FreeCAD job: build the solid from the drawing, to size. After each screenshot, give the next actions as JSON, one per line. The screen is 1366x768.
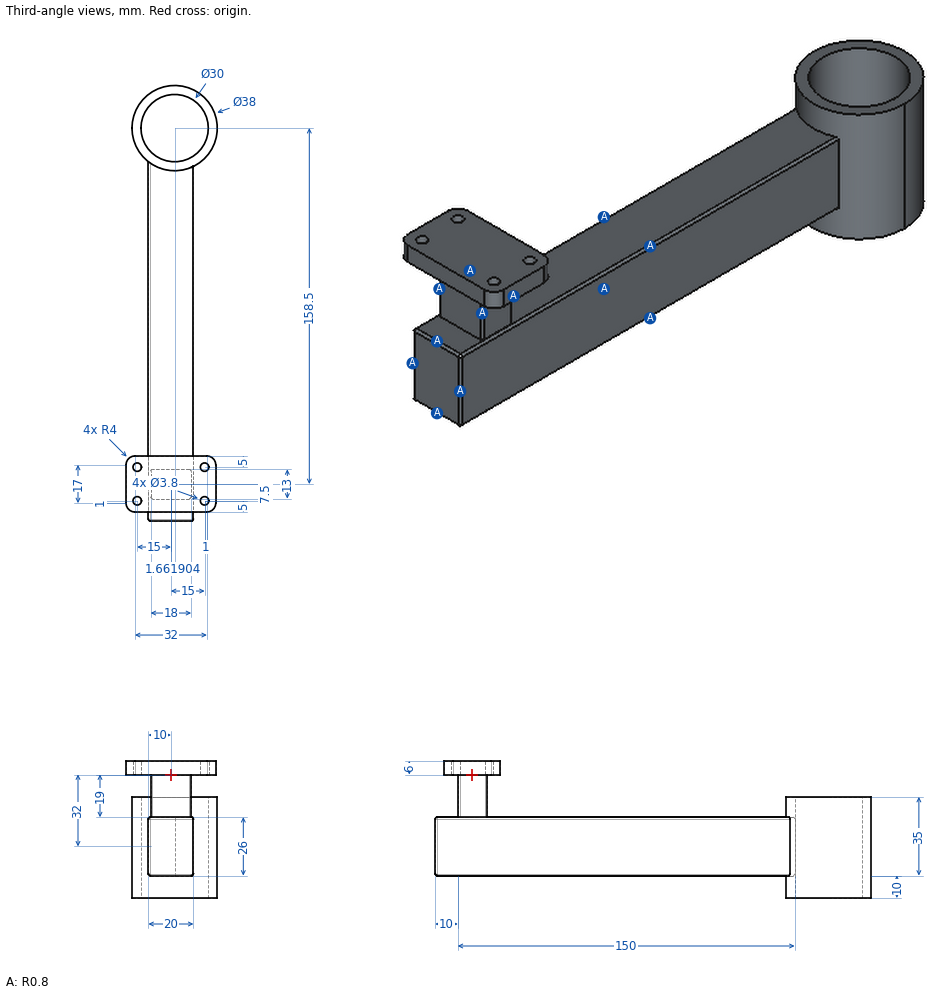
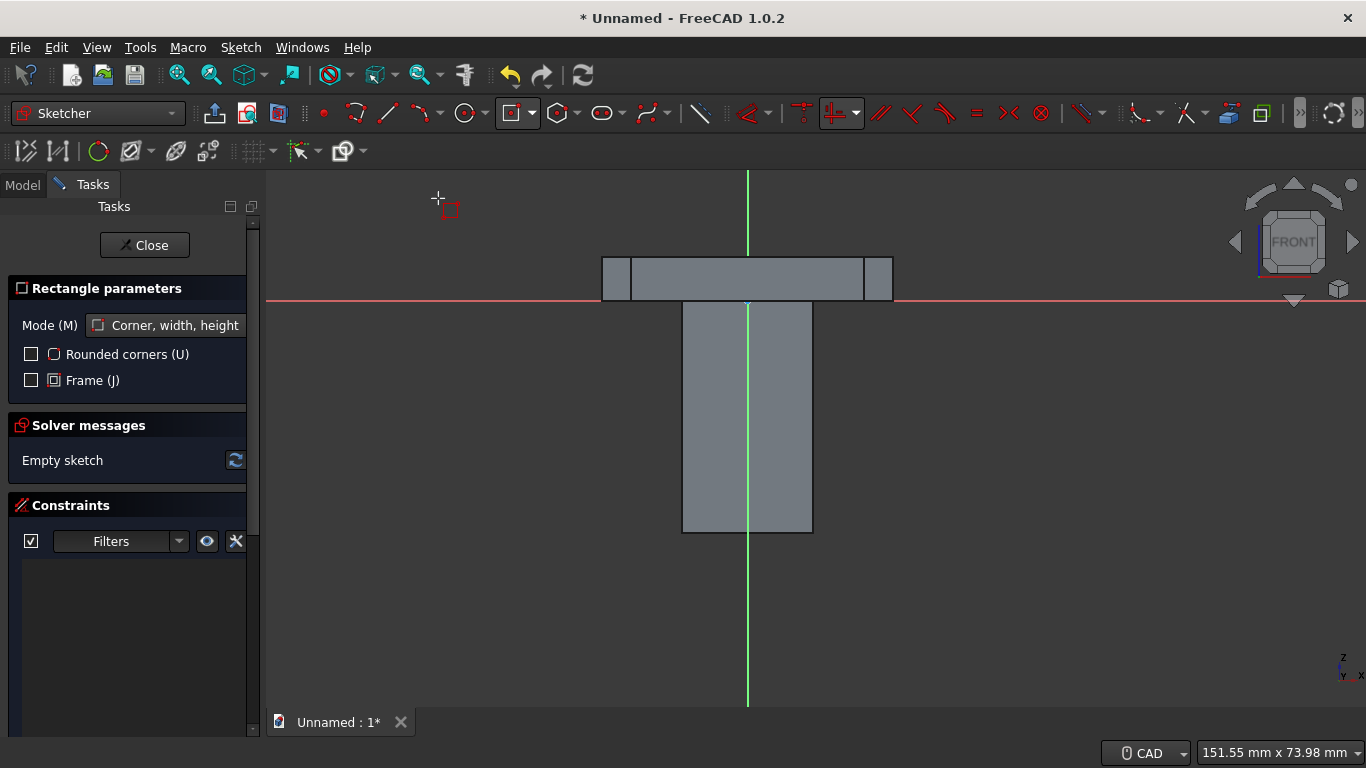
{"action": "left_click", "coordinate": [675, 438]}
{"action": "mouse_move", "coordinate": [820, 627]}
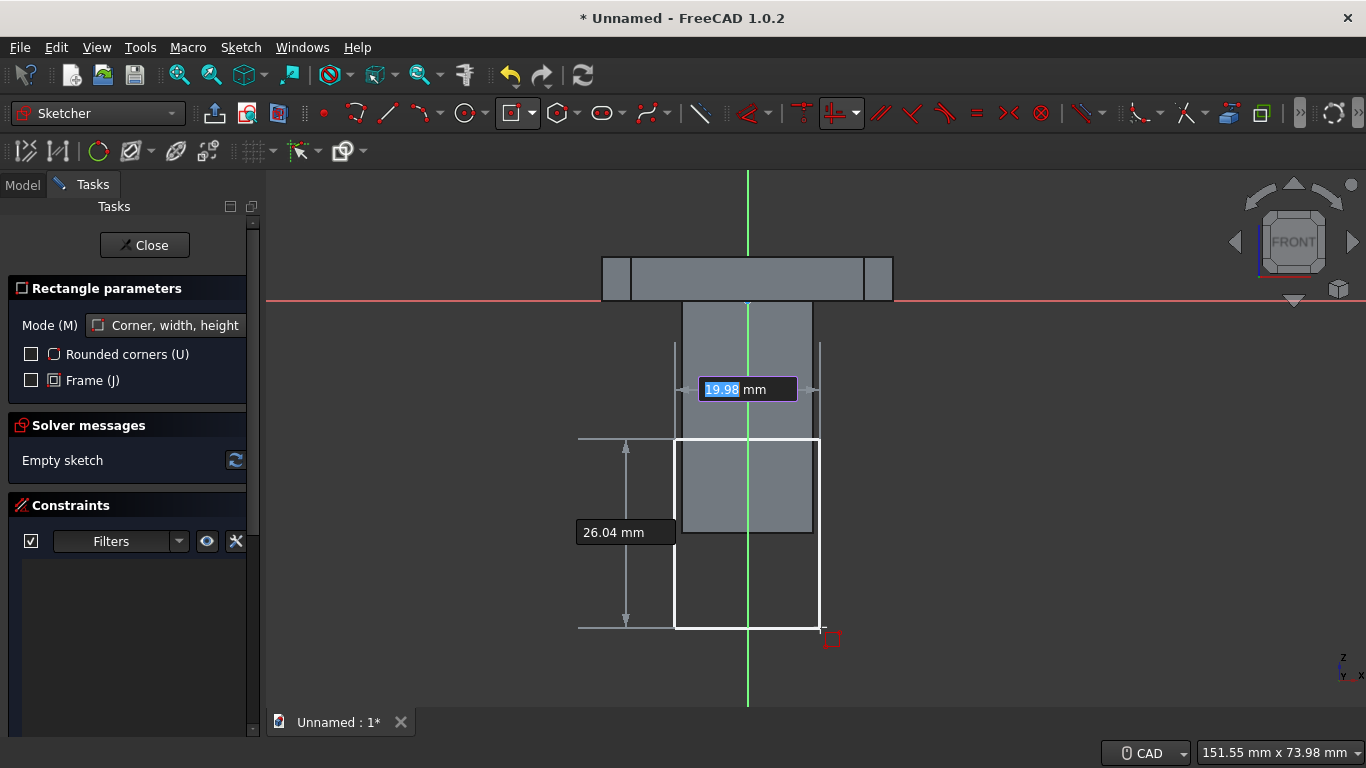
{"action": "type", "text": "20"}
{"action": "key", "text": "Tab"}
{"action": "type", "text": "26"}
{"action": "key", "text": "Return"}
{"action": "key", "text": "Escape"}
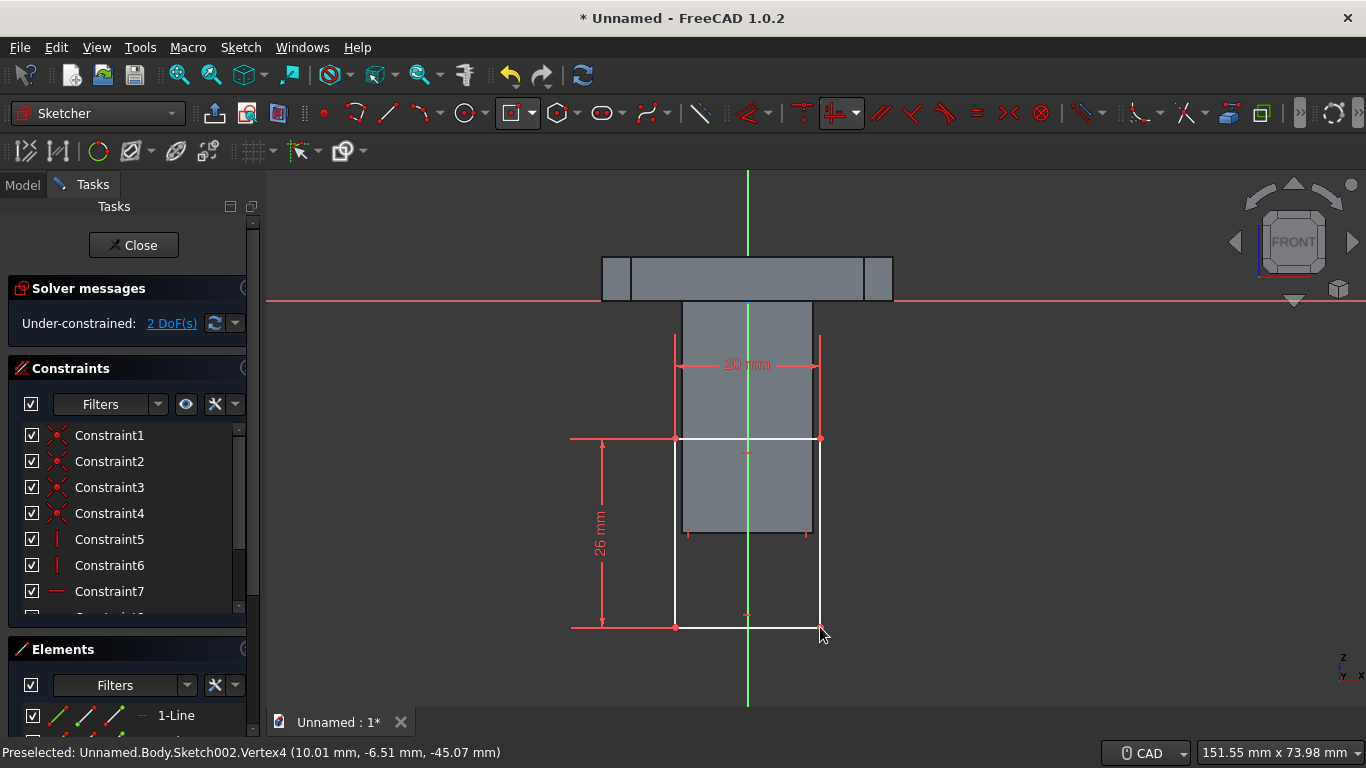
{"action": "left_click", "coordinate": [748, 114]}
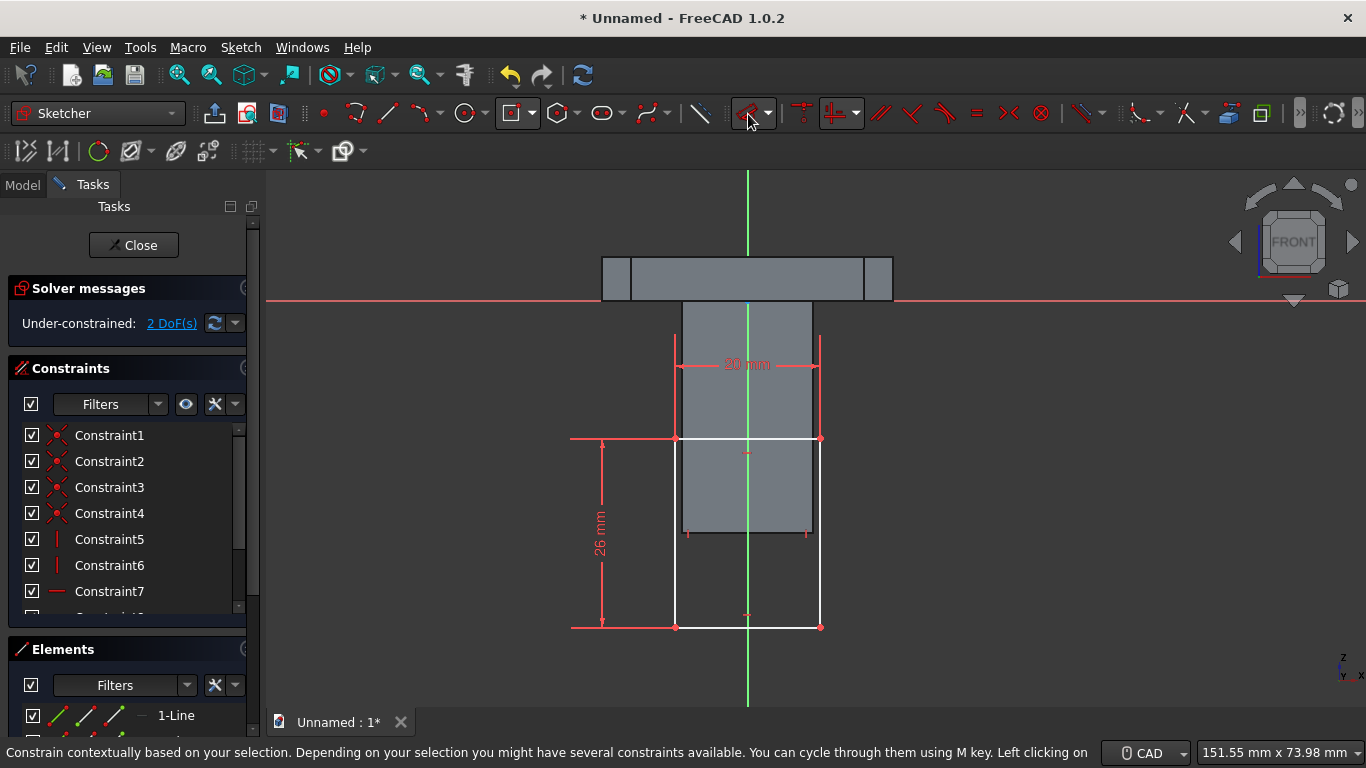
{"action": "left_click", "coordinate": [675, 439]}
{"action": "left_click", "coordinate": [711, 267]}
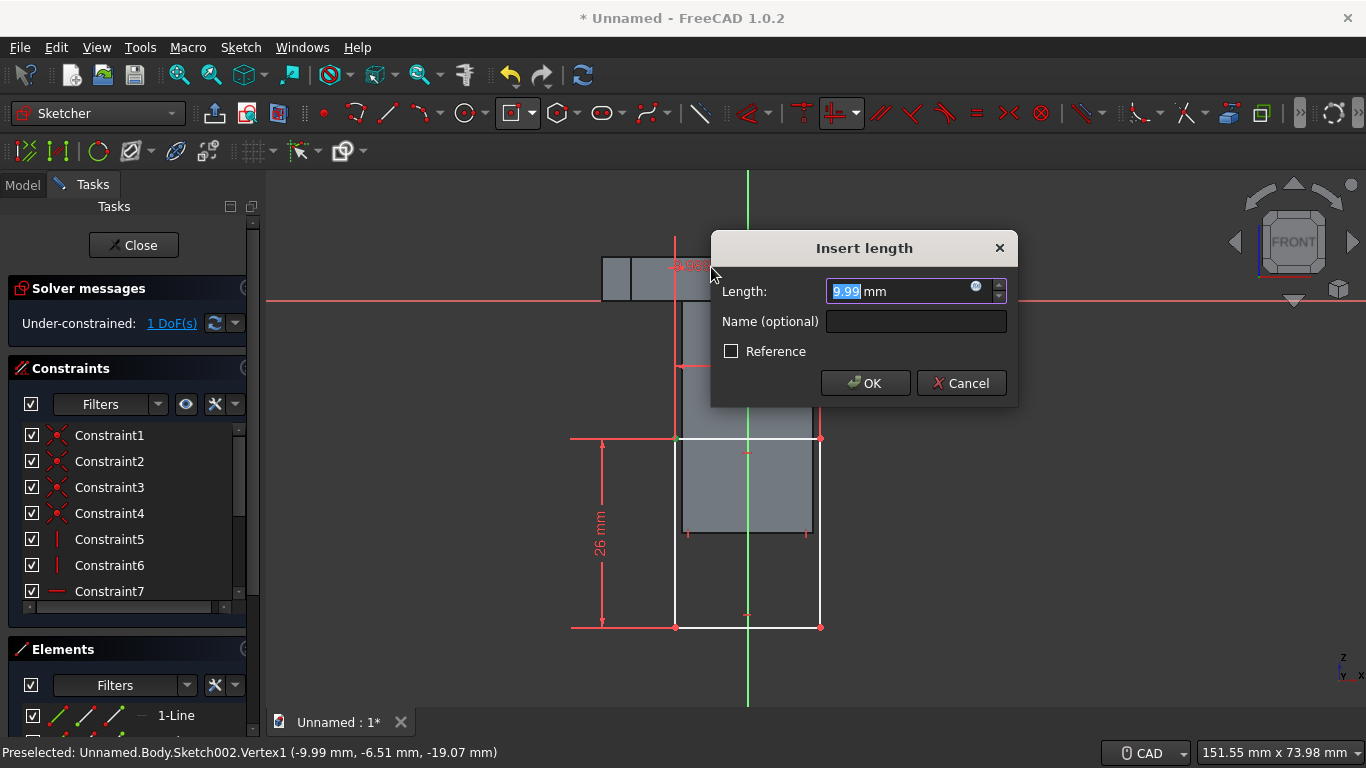
{"action": "type", "text": "10"}
{"action": "key", "text": "Return"}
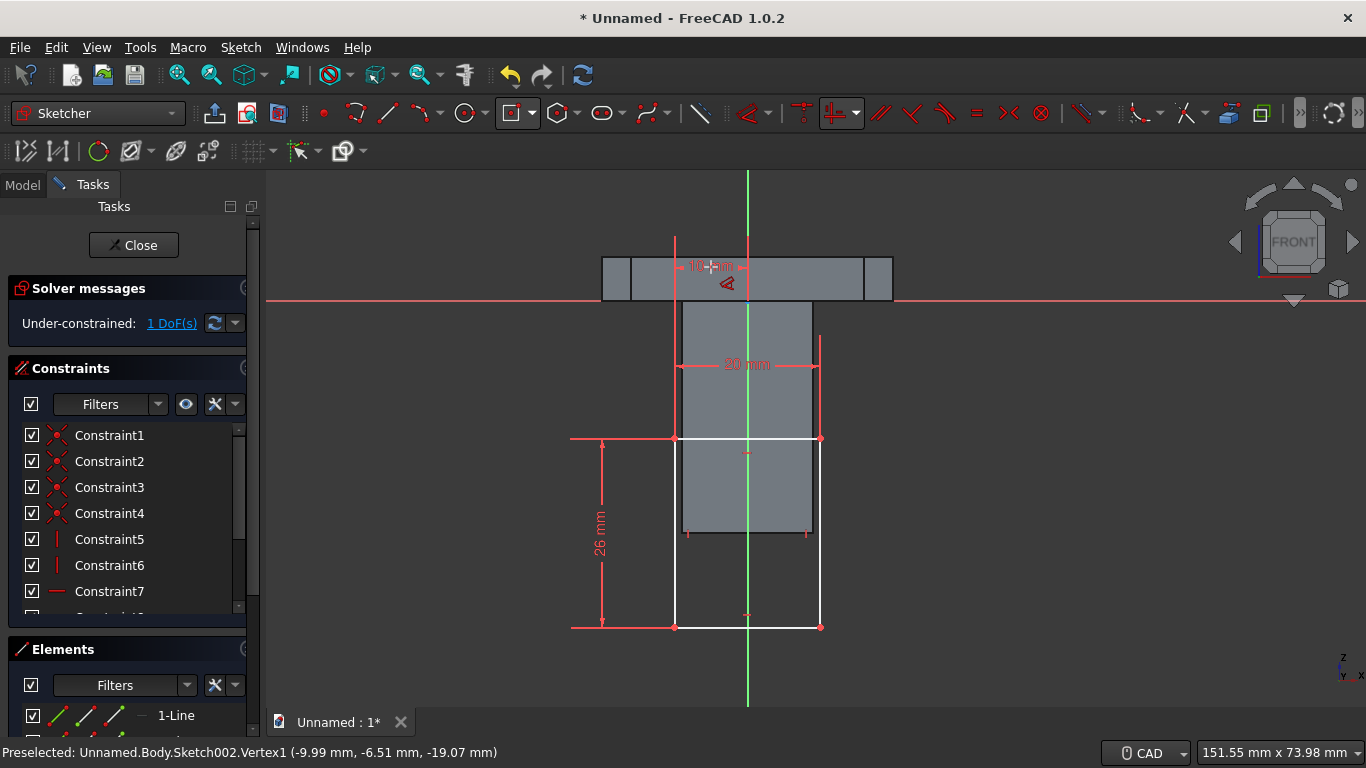
{"action": "left_click", "coordinate": [675, 439]}
{"action": "left_click", "coordinate": [641, 370]}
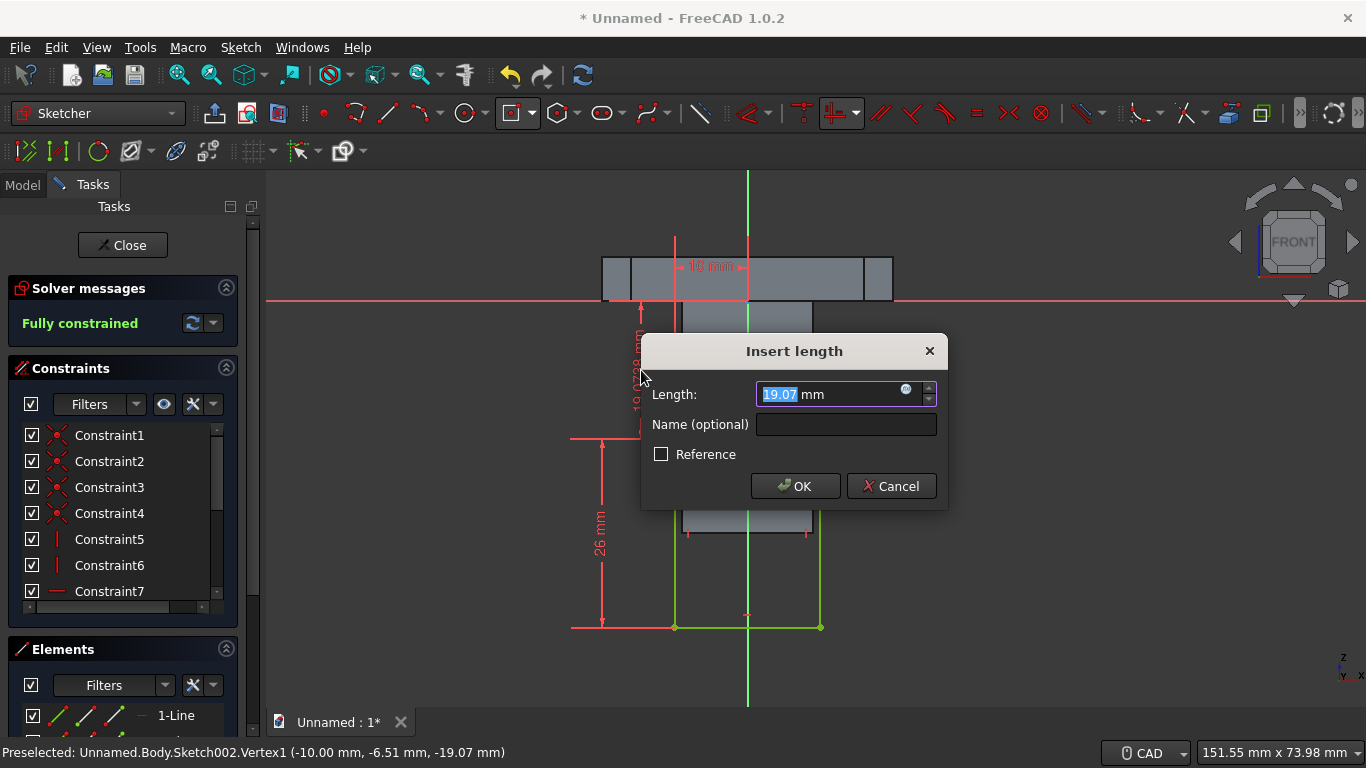
{"action": "type", "text": "19"}
{"action": "key", "text": "Return"}
{"action": "key", "text": "Escape"}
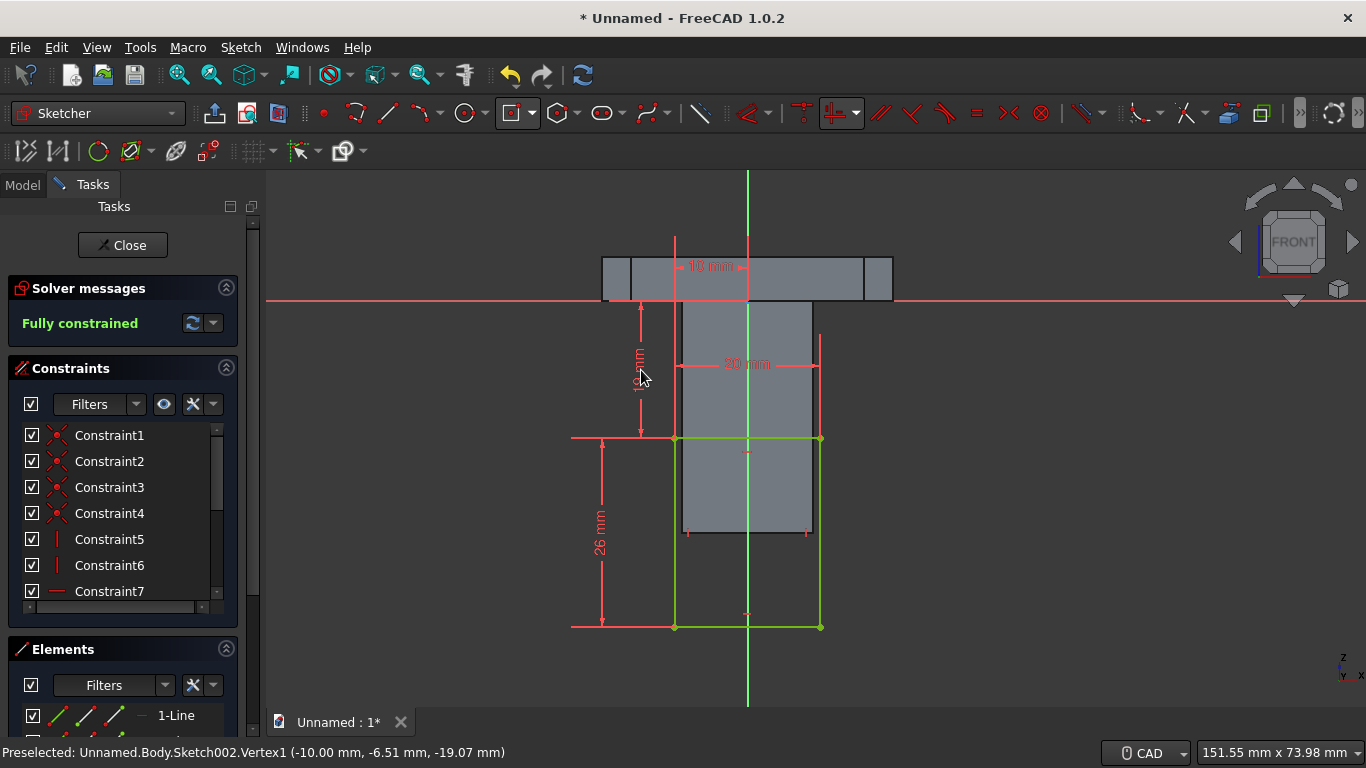
{"action": "left_click", "coordinate": [123, 245]}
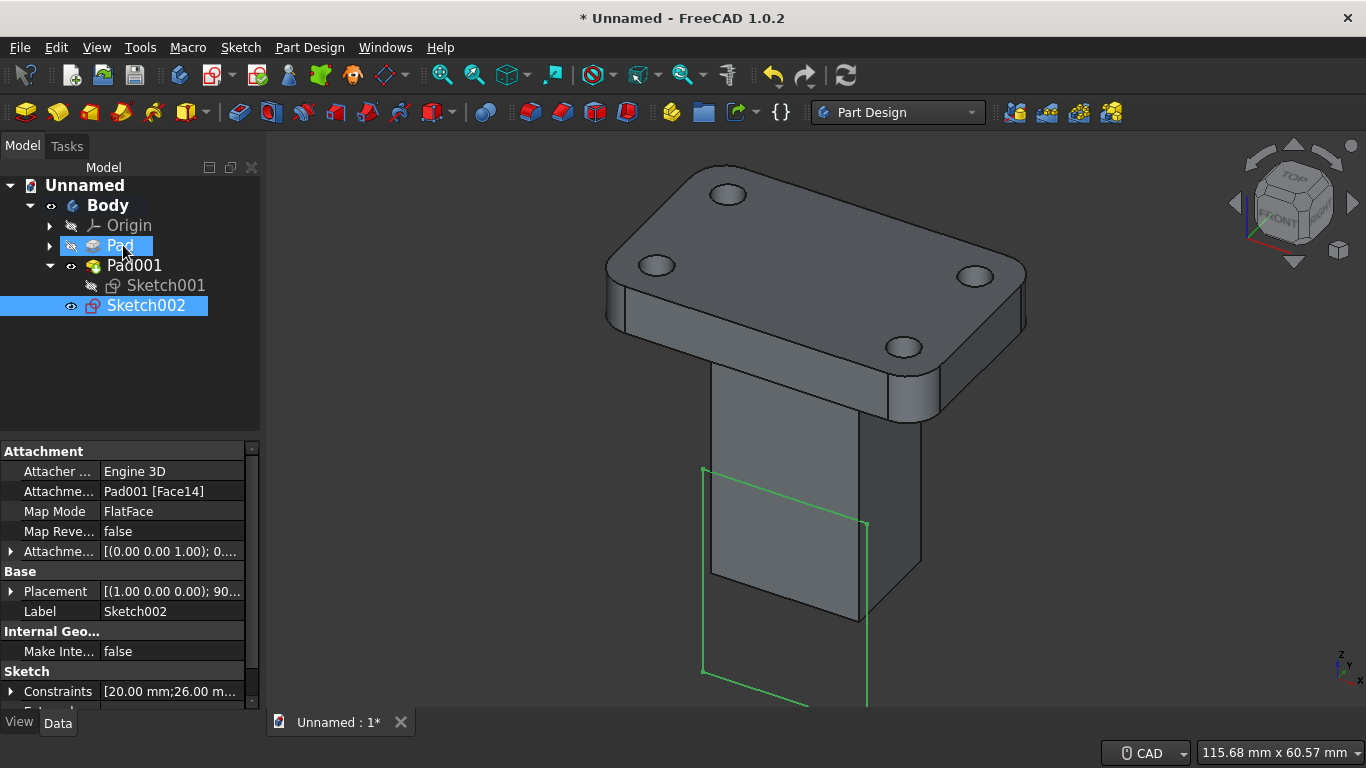
{"action": "left_click", "coordinate": [26, 112]}